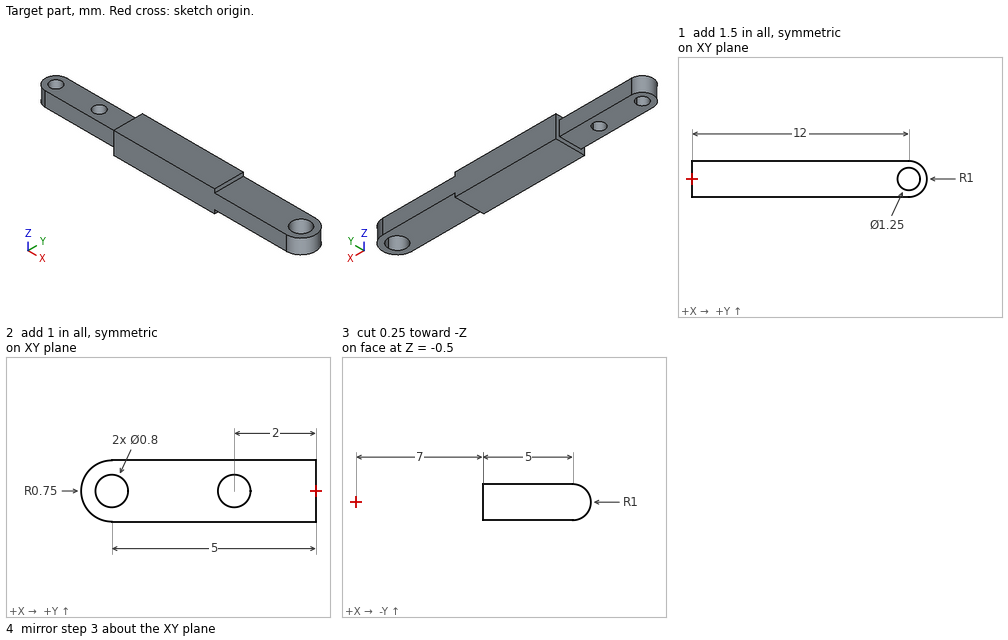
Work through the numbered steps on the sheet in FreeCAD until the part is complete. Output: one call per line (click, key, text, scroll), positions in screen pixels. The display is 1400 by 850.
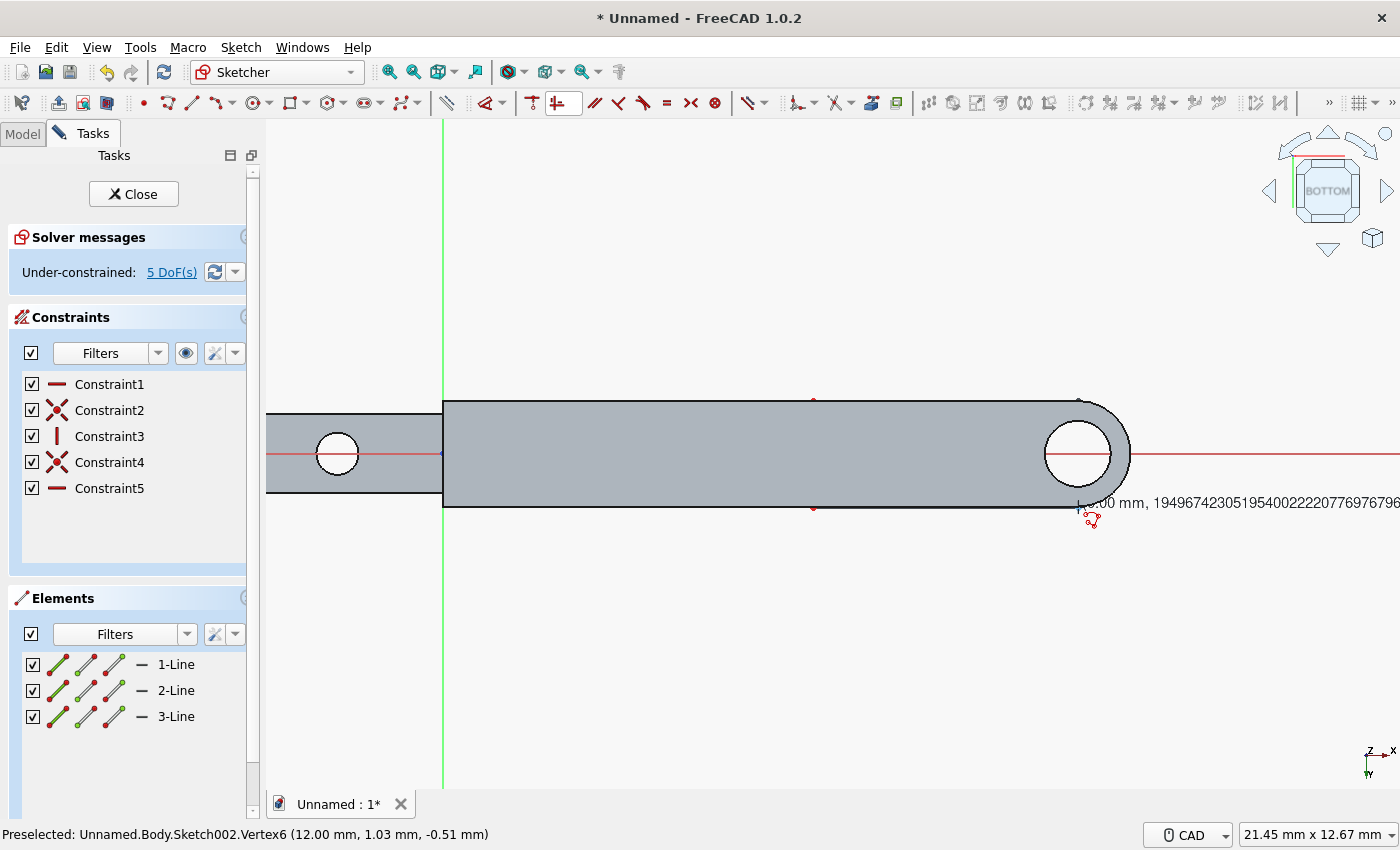
click(216, 104)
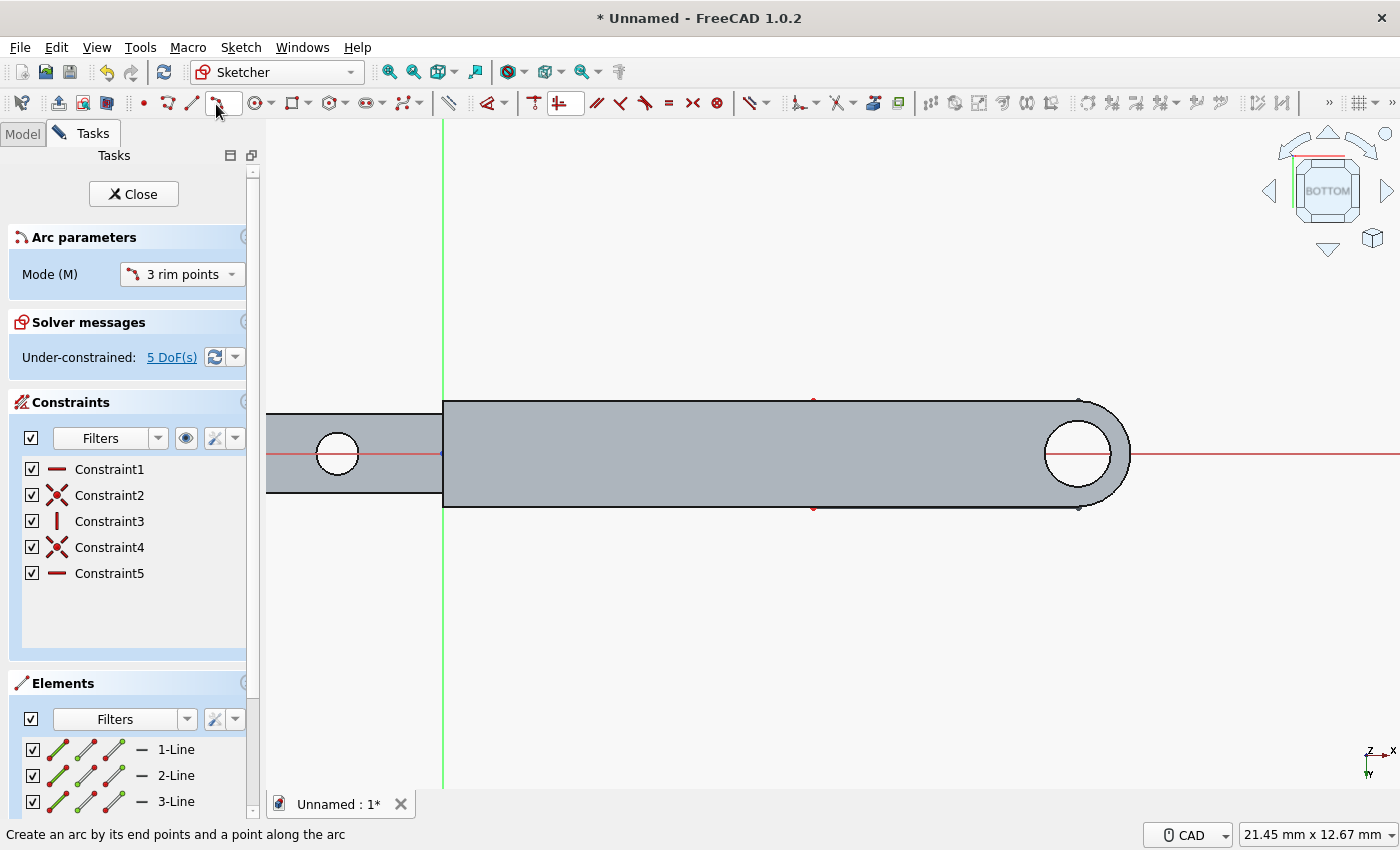
click(1078, 508)
click(1078, 402)
click(1128, 470)
key(Escape)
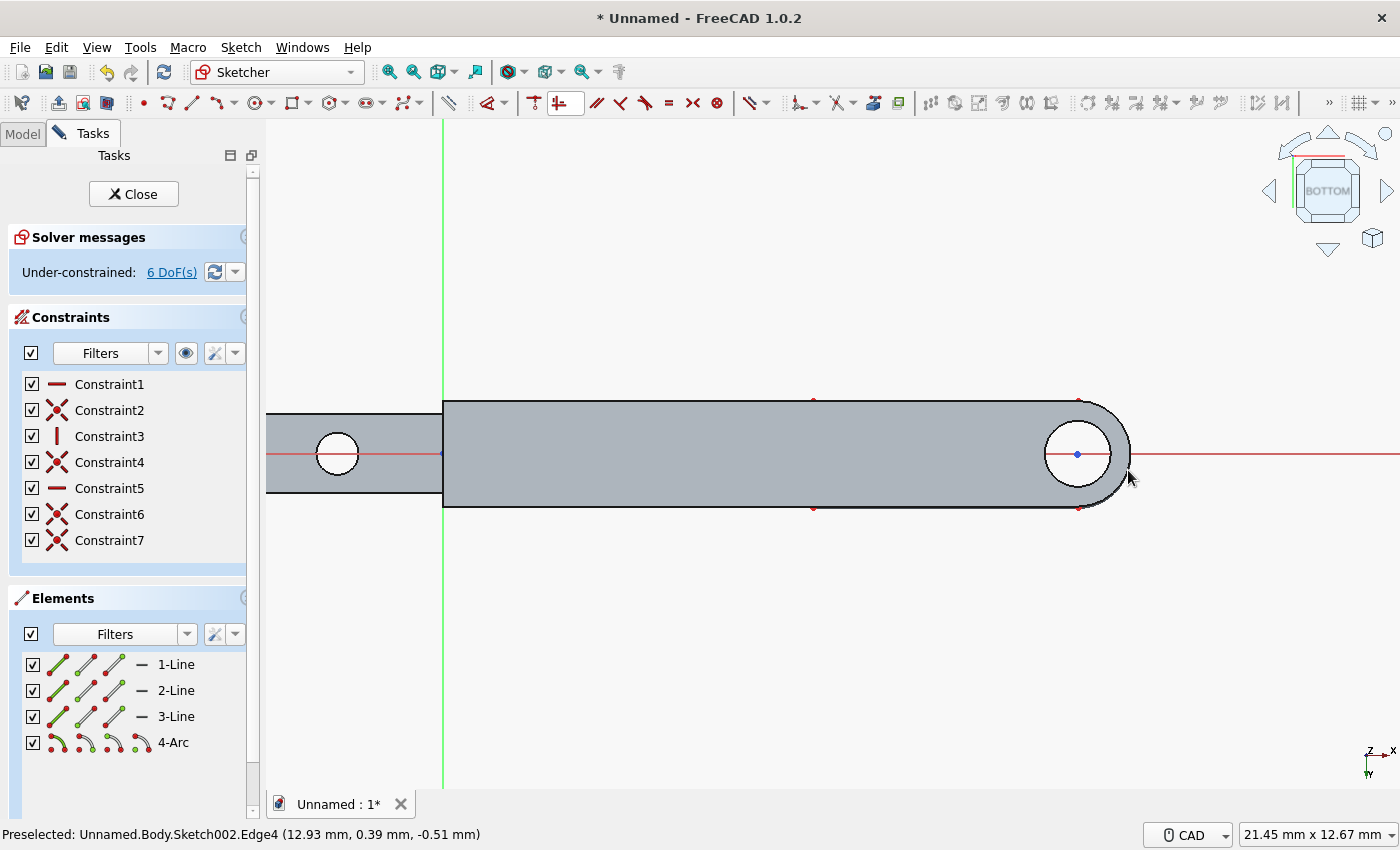
click(998, 402)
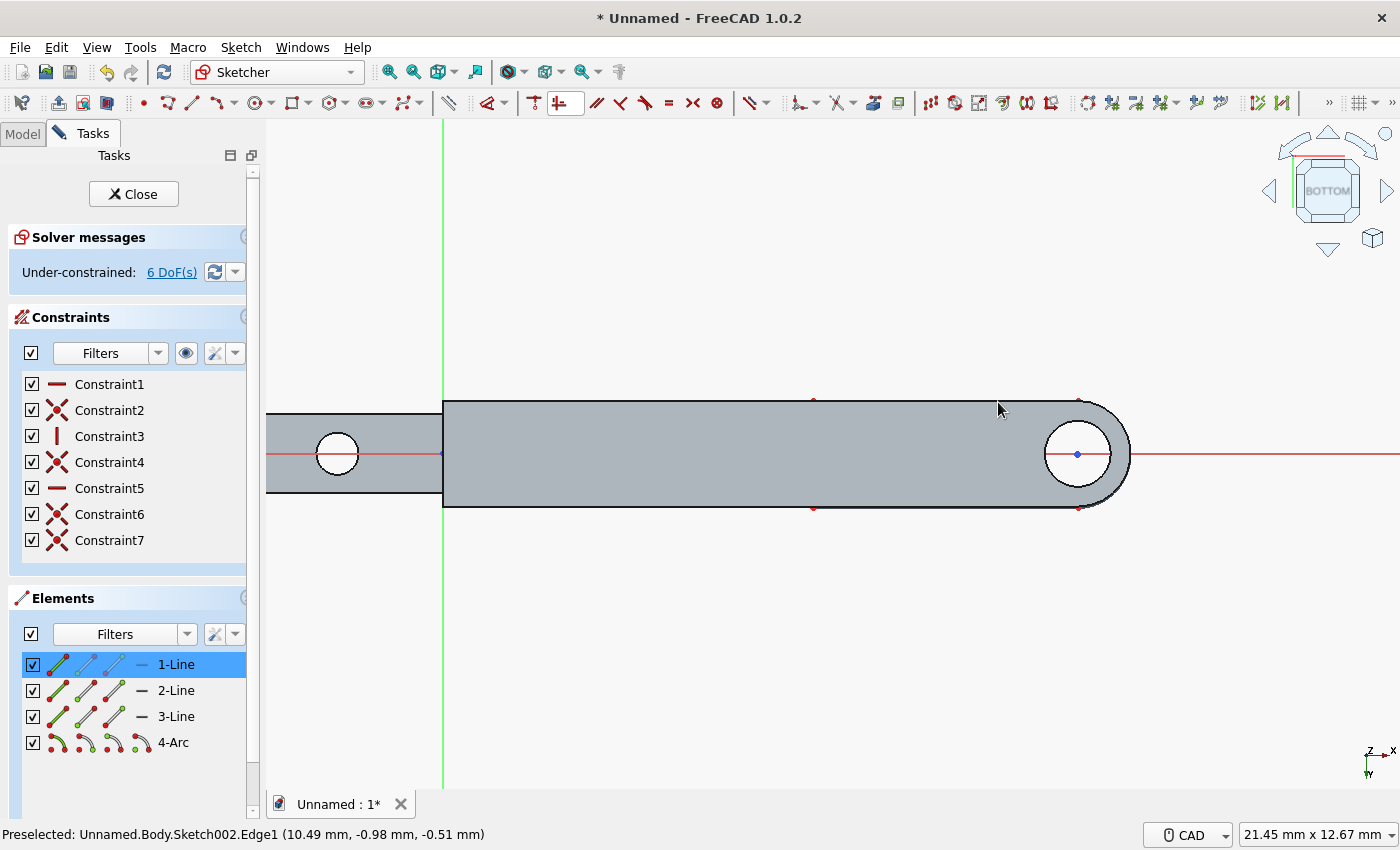
click(1120, 486)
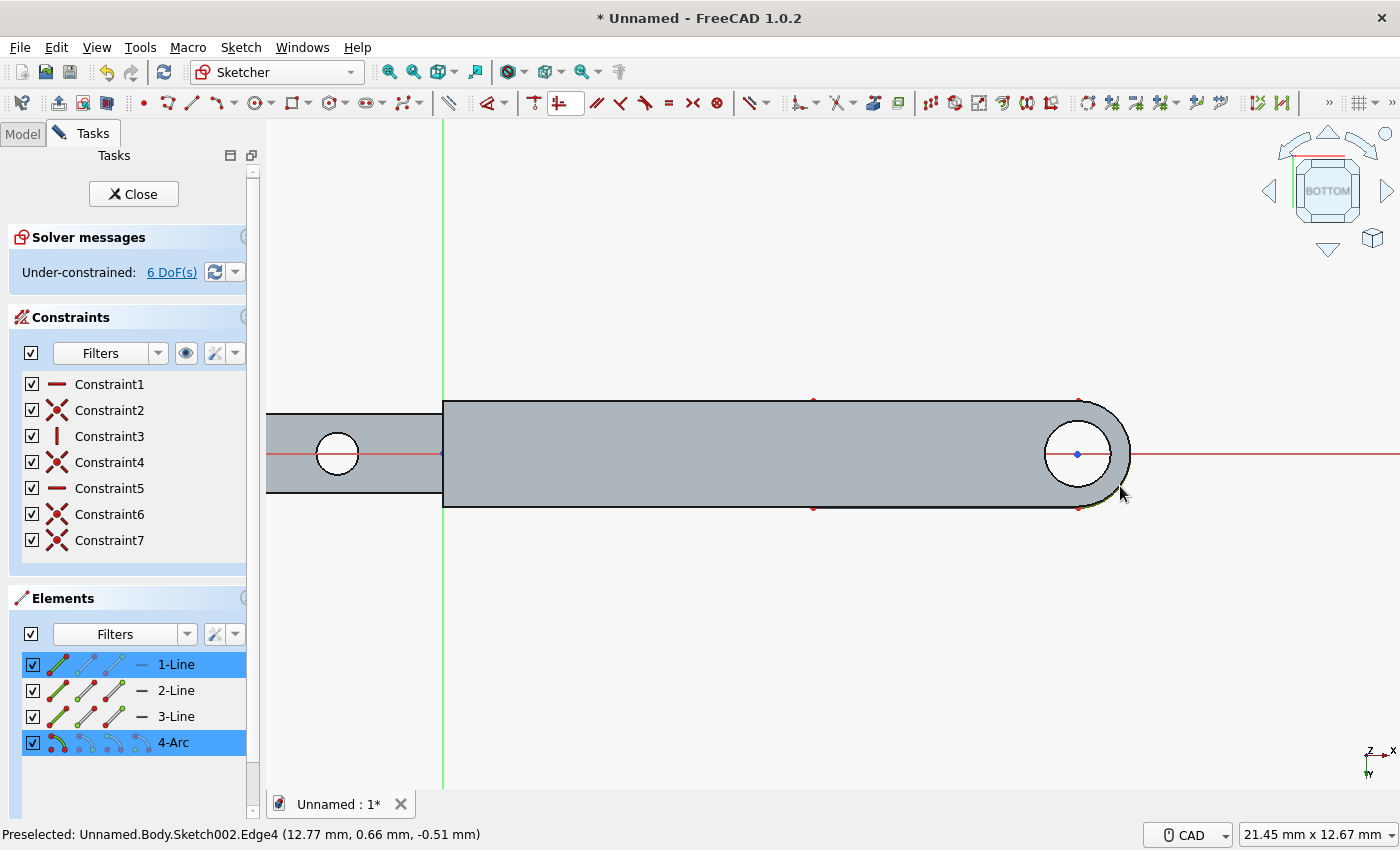
click(646, 104)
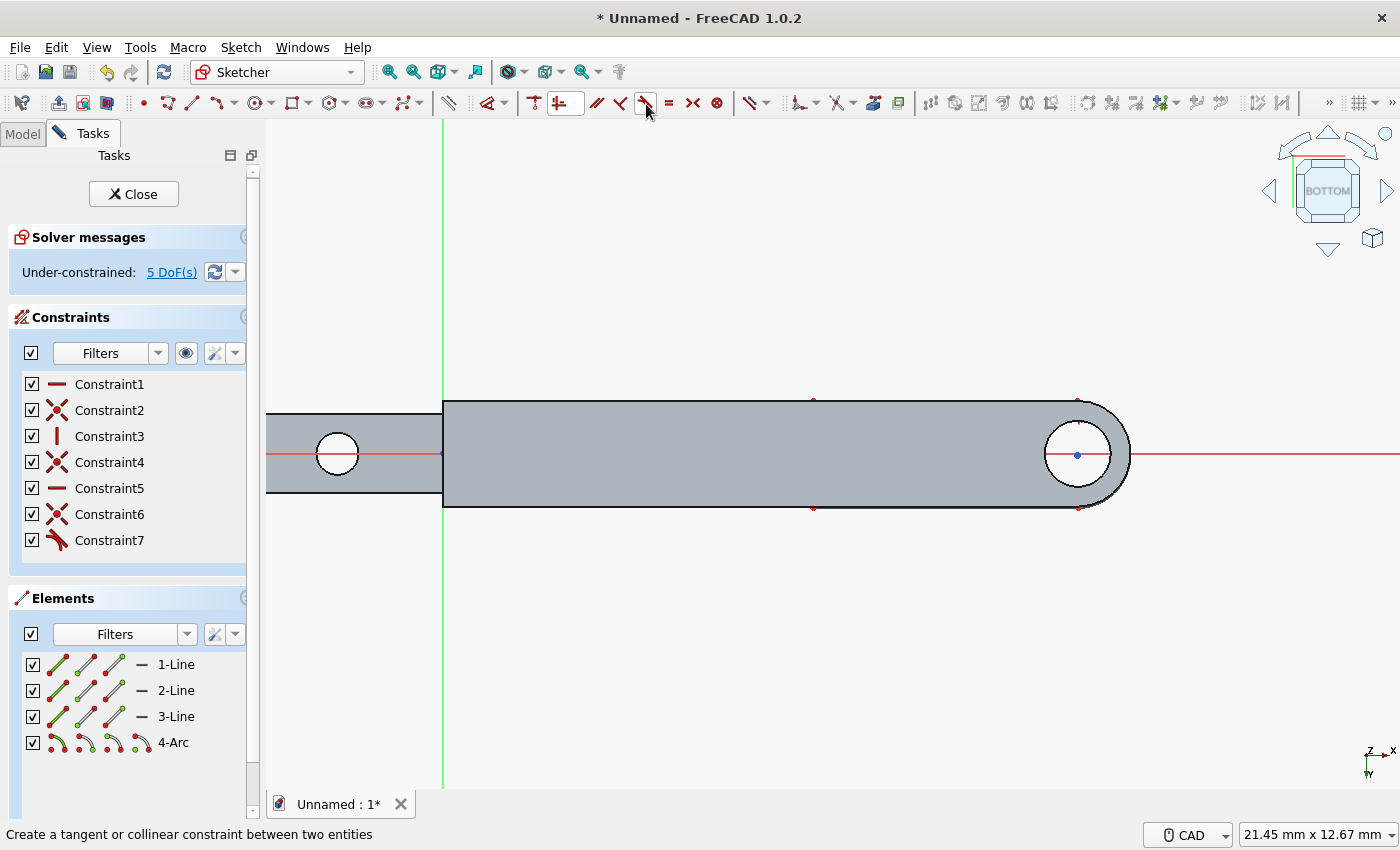
click(892, 508)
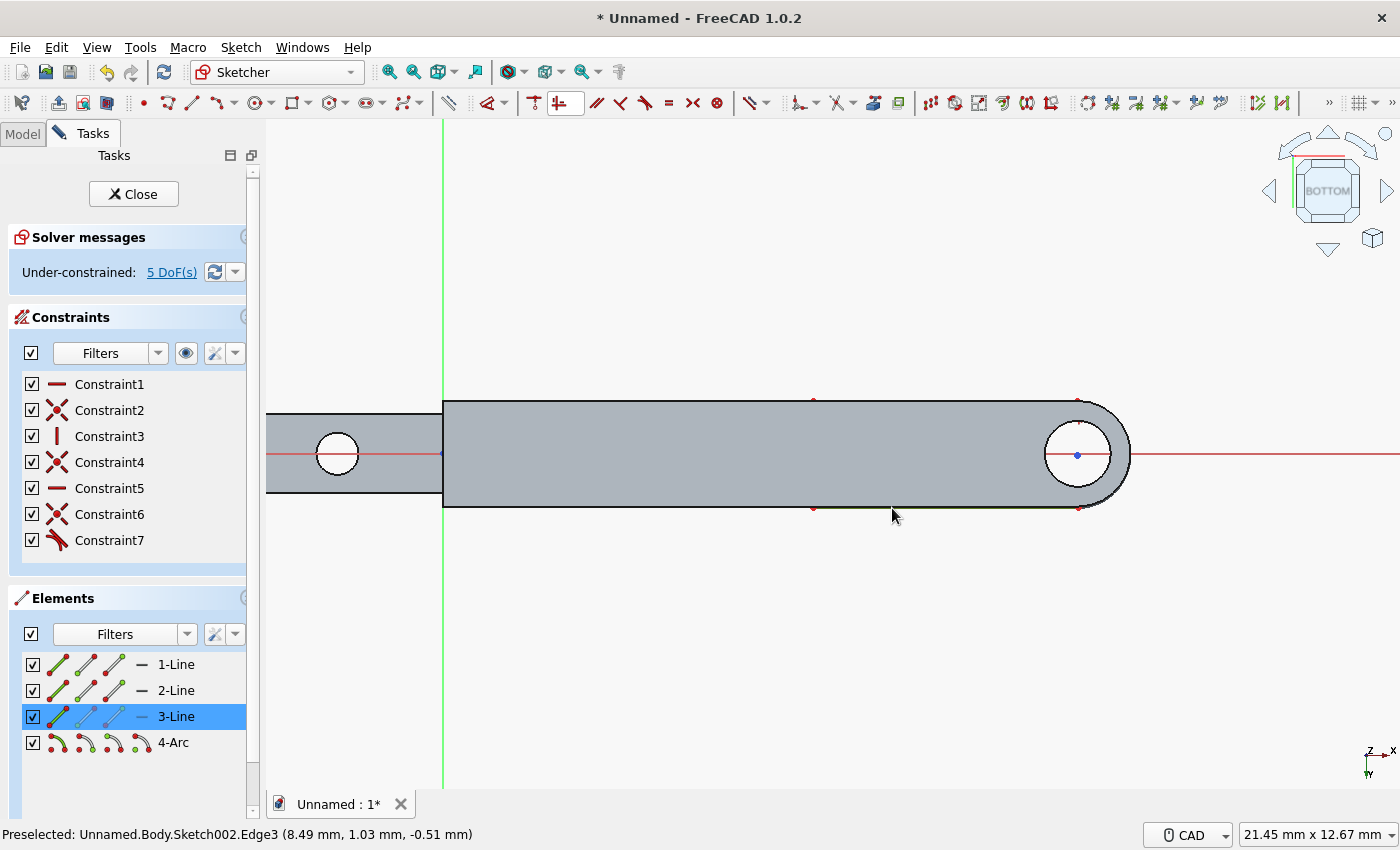
click(1121, 486)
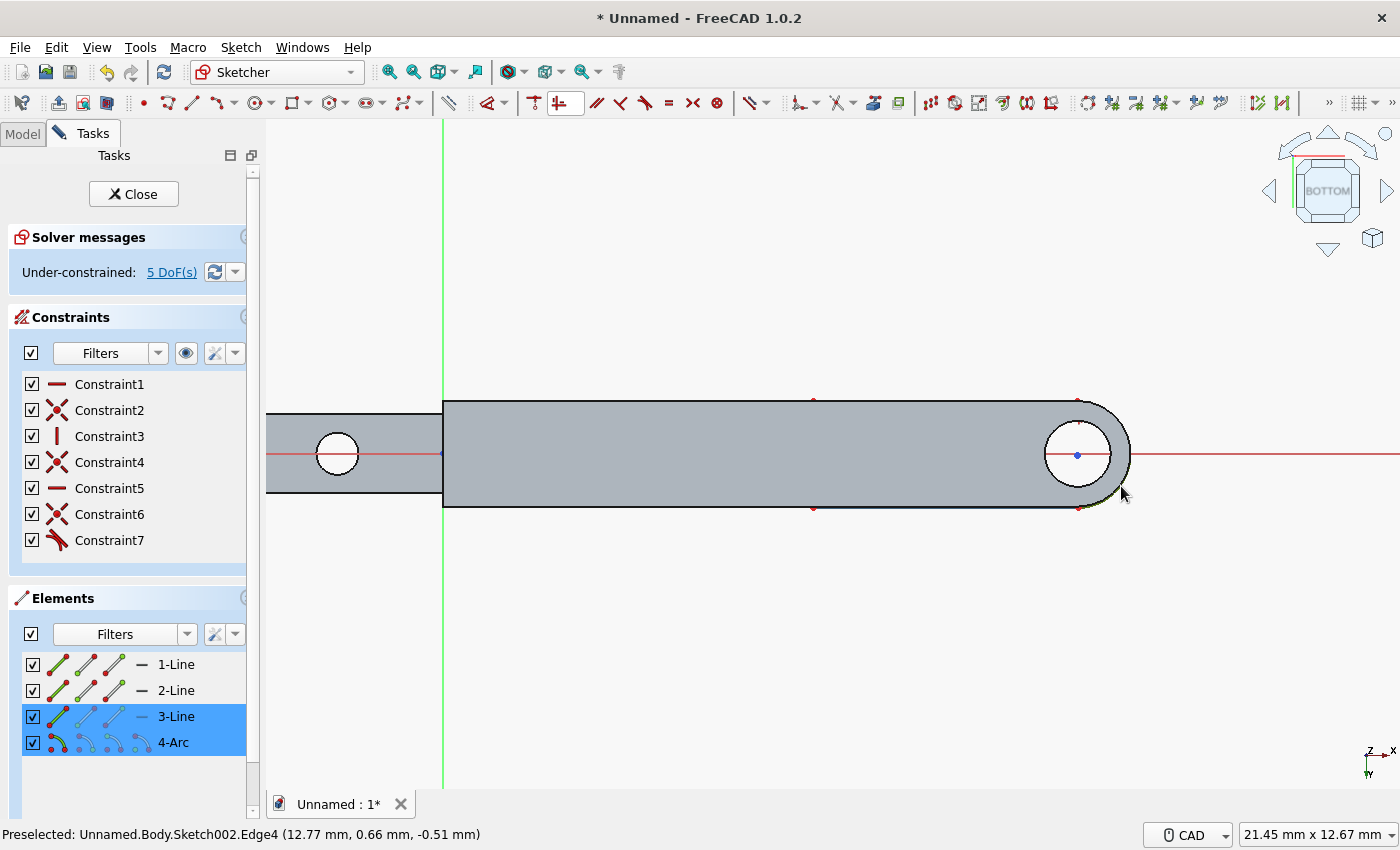
click(646, 104)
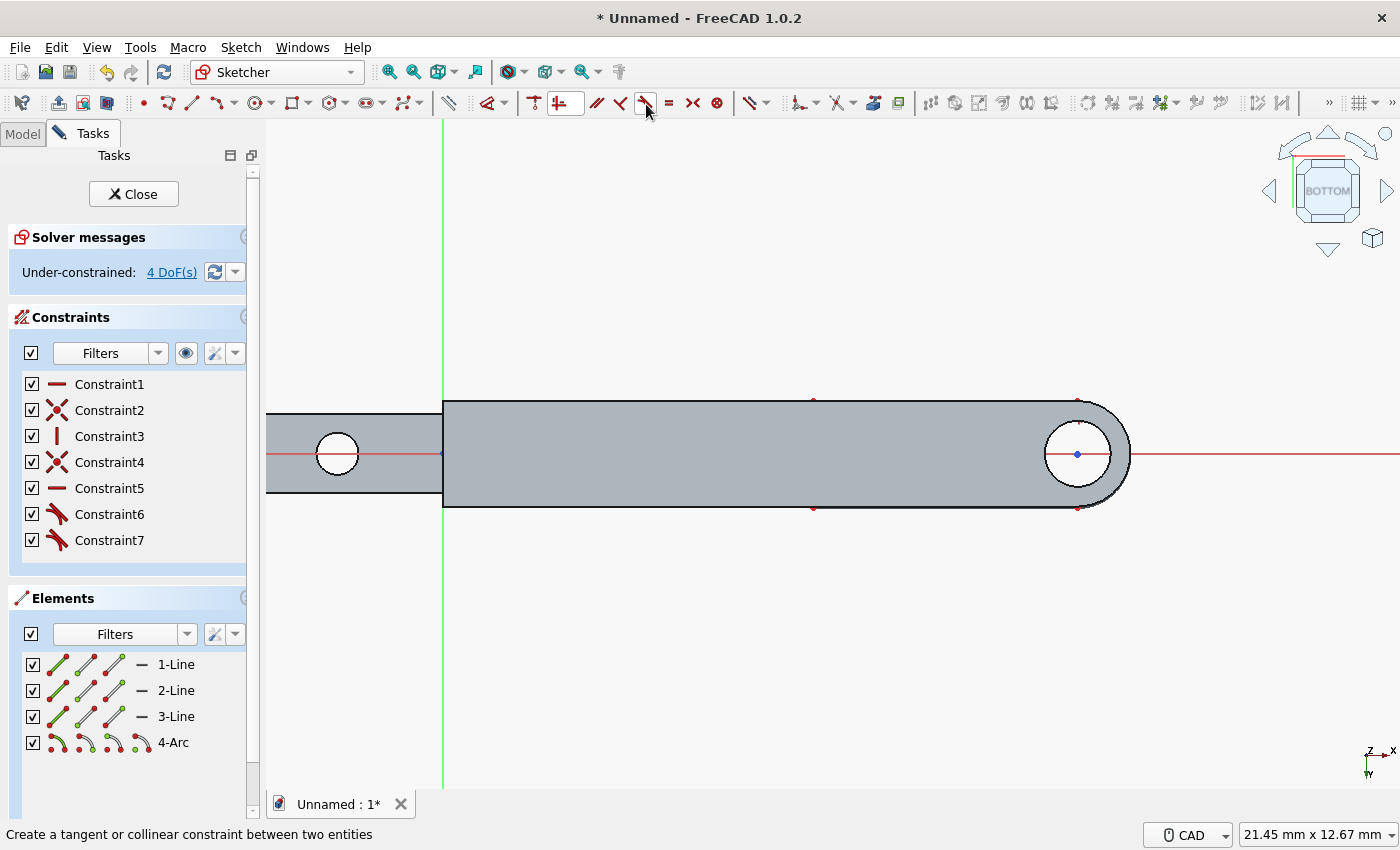
click(1077, 455)